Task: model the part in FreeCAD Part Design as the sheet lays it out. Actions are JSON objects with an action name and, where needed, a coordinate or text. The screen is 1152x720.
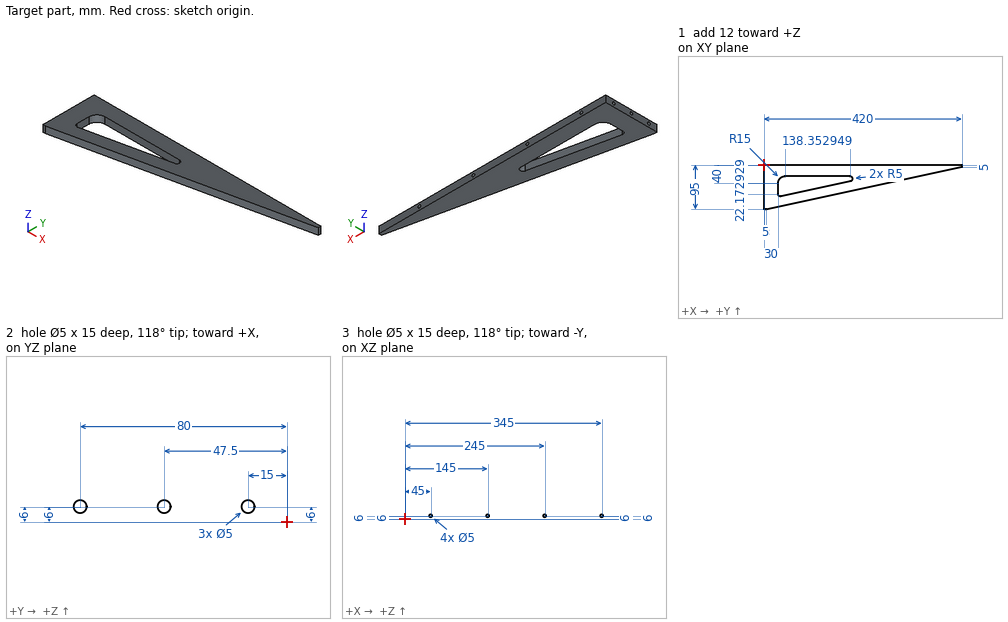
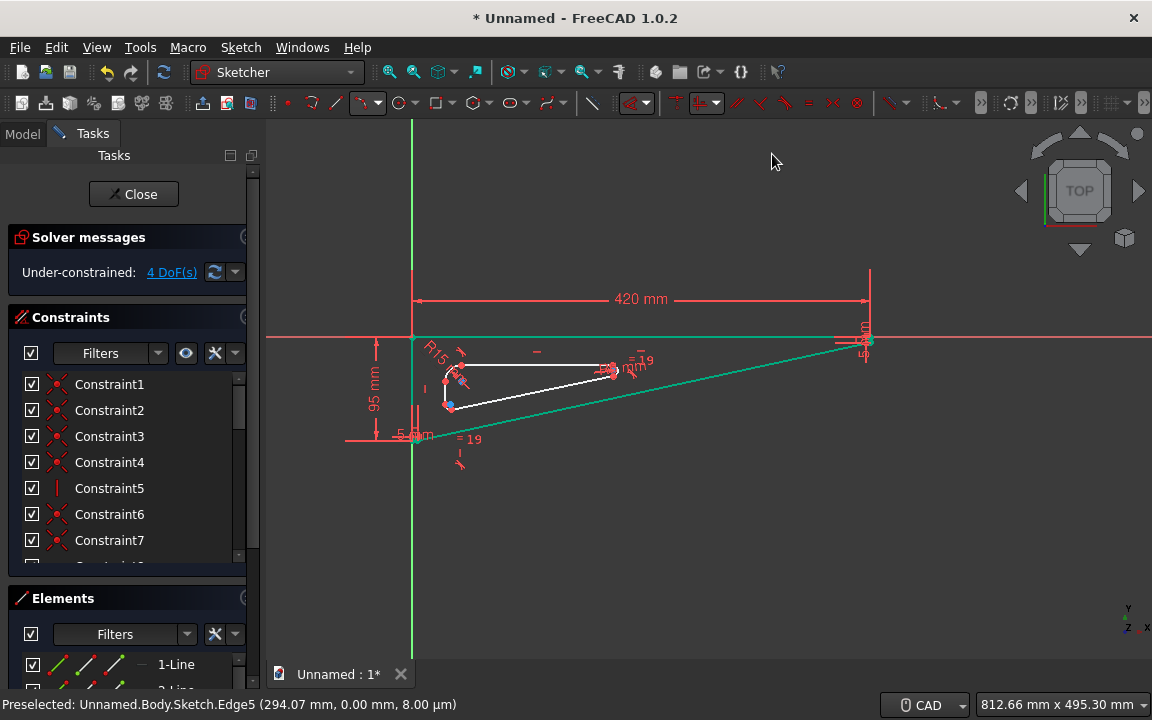
{"action": "scroll", "coordinate": [445, 405], "scroll_direction": "up", "scroll_amount": 5}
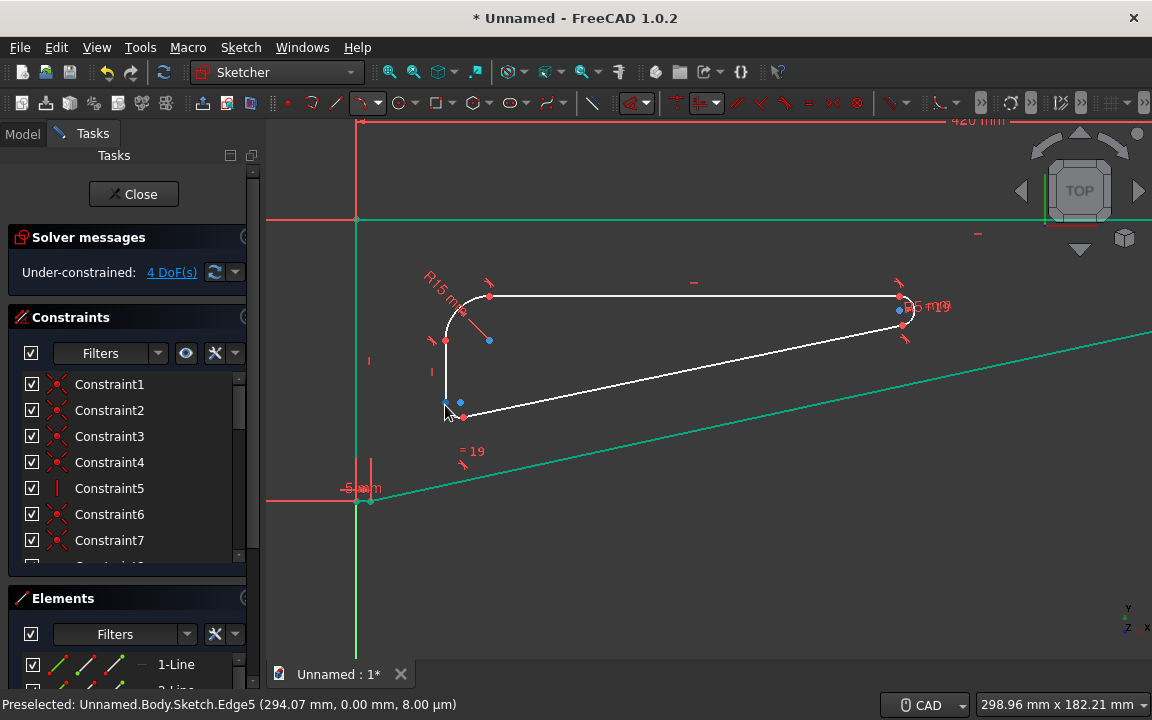
{"action": "left_click", "coordinate": [446, 403]}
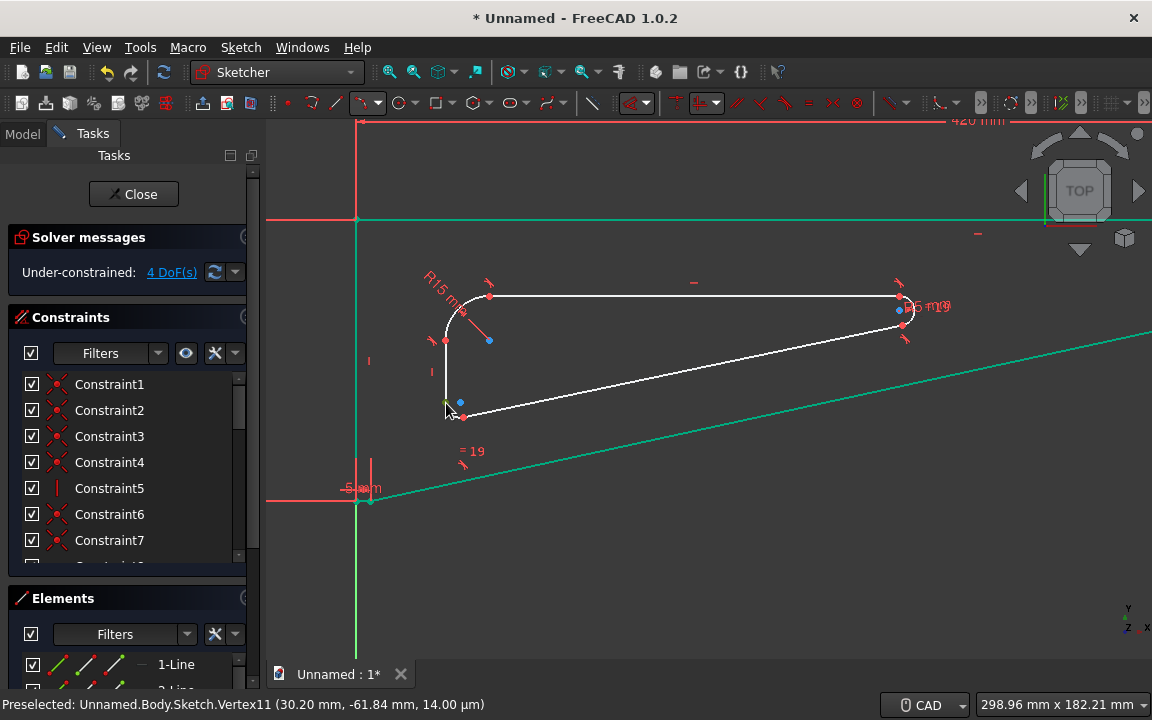
{"action": "left_click", "coordinate": [648, 104]}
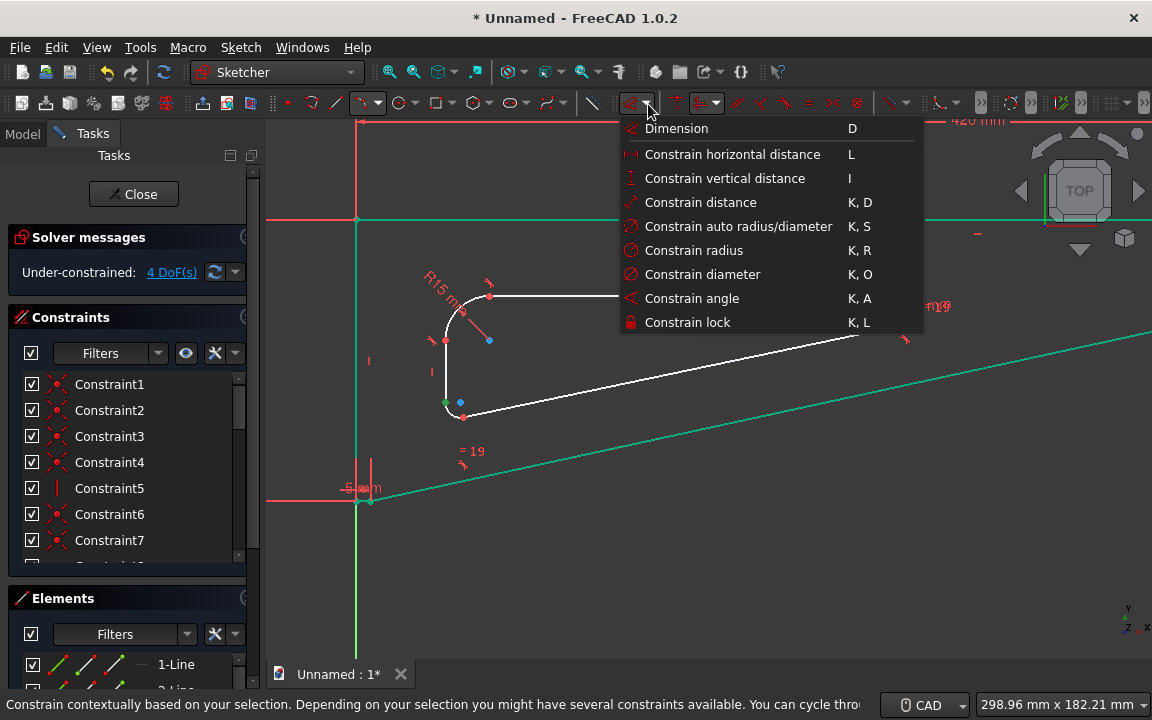
{"action": "left_click", "coordinate": [772, 154]}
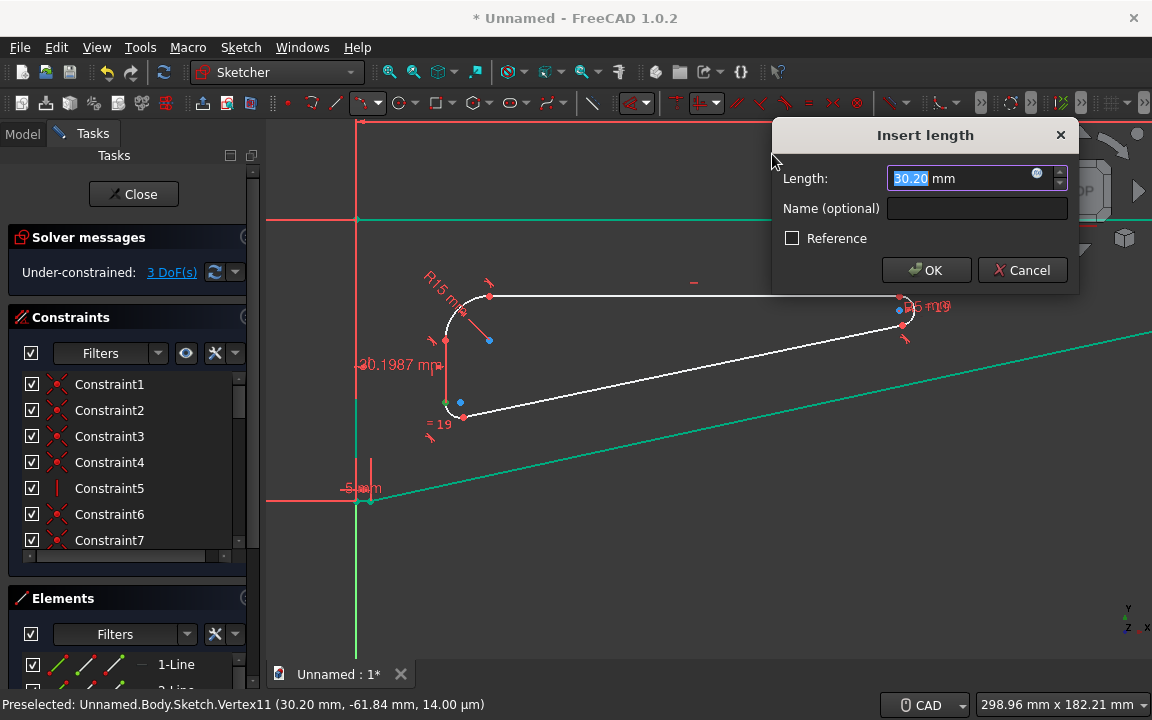
{"action": "type", "text": "30"}
{"action": "key", "text": "Return"}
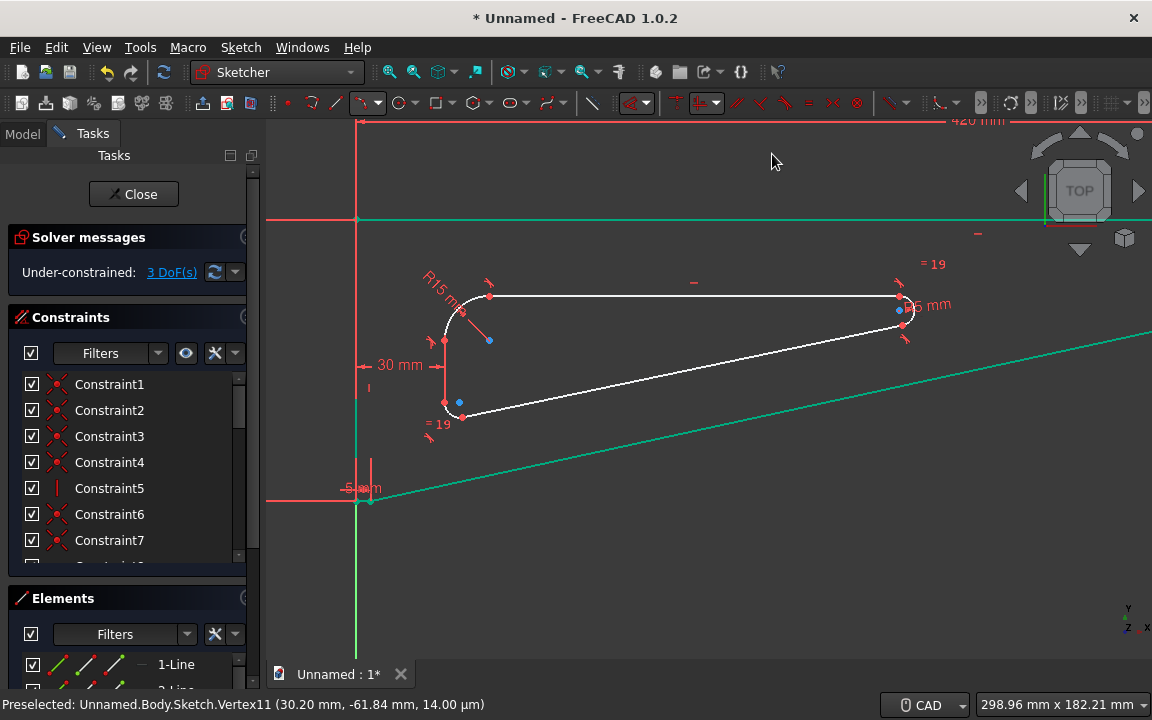
{"action": "left_click", "coordinate": [445, 340]}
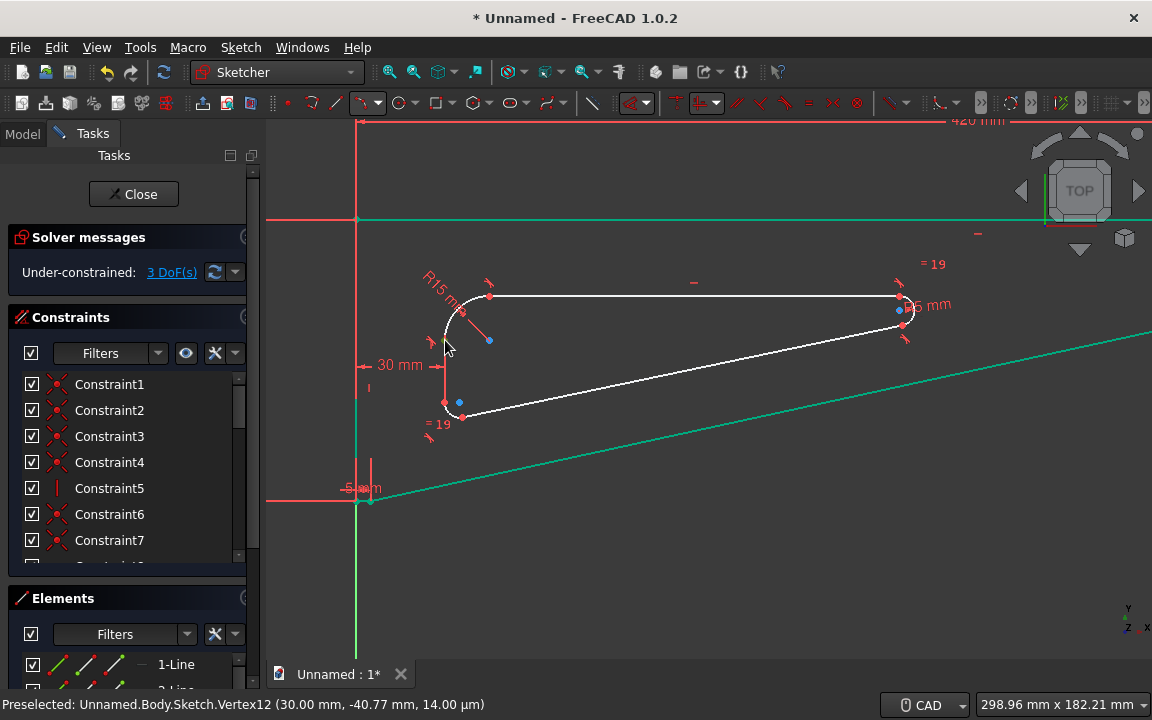
{"action": "key", "text": "i"}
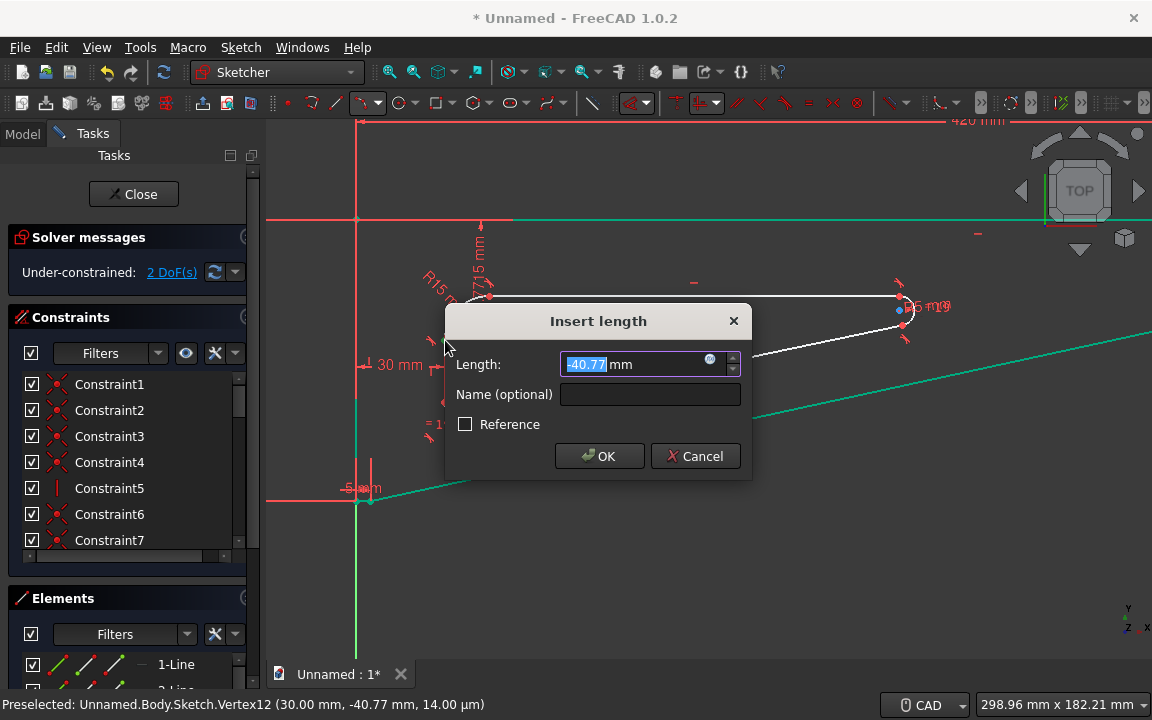
{"action": "type", "text": "-40"}
{"action": "key", "text": "Return"}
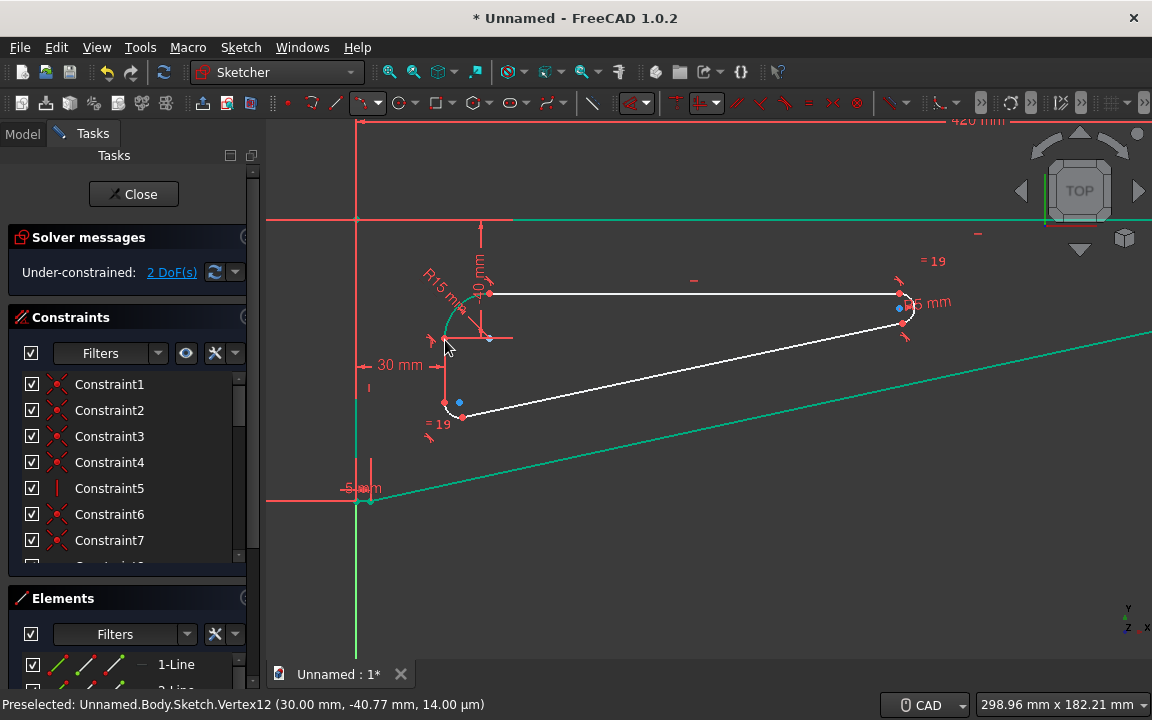
{"action": "left_click", "coordinate": [445, 383]}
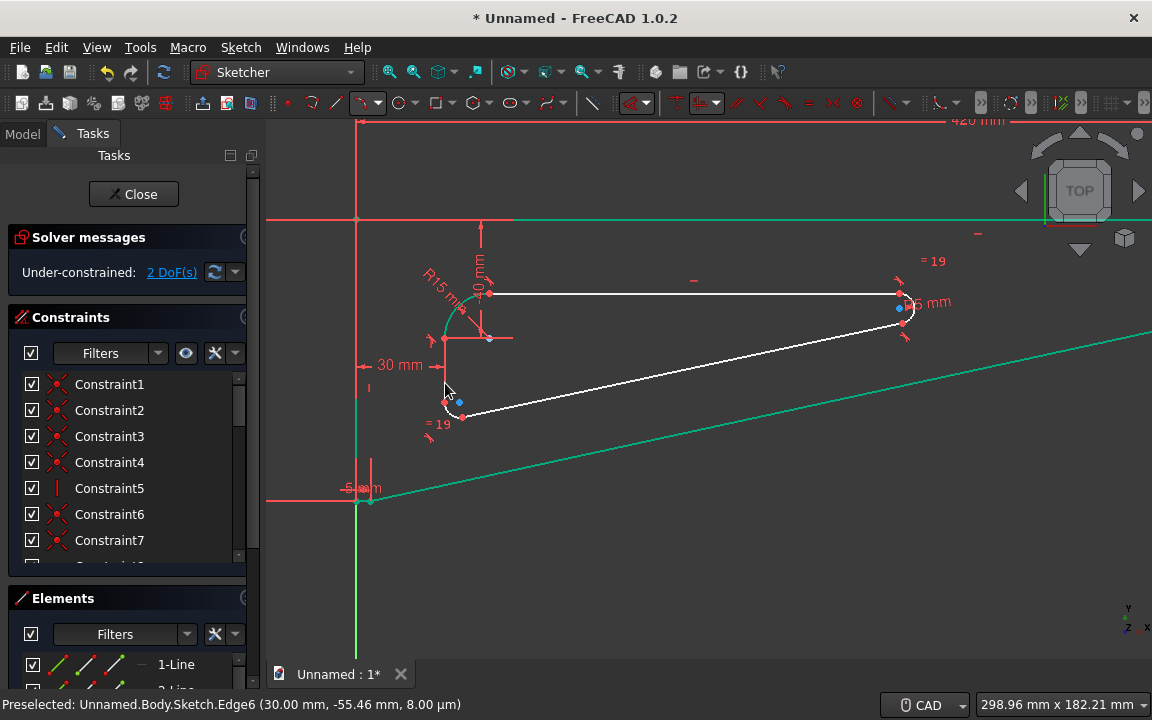
{"action": "left_click", "coordinate": [648, 104]}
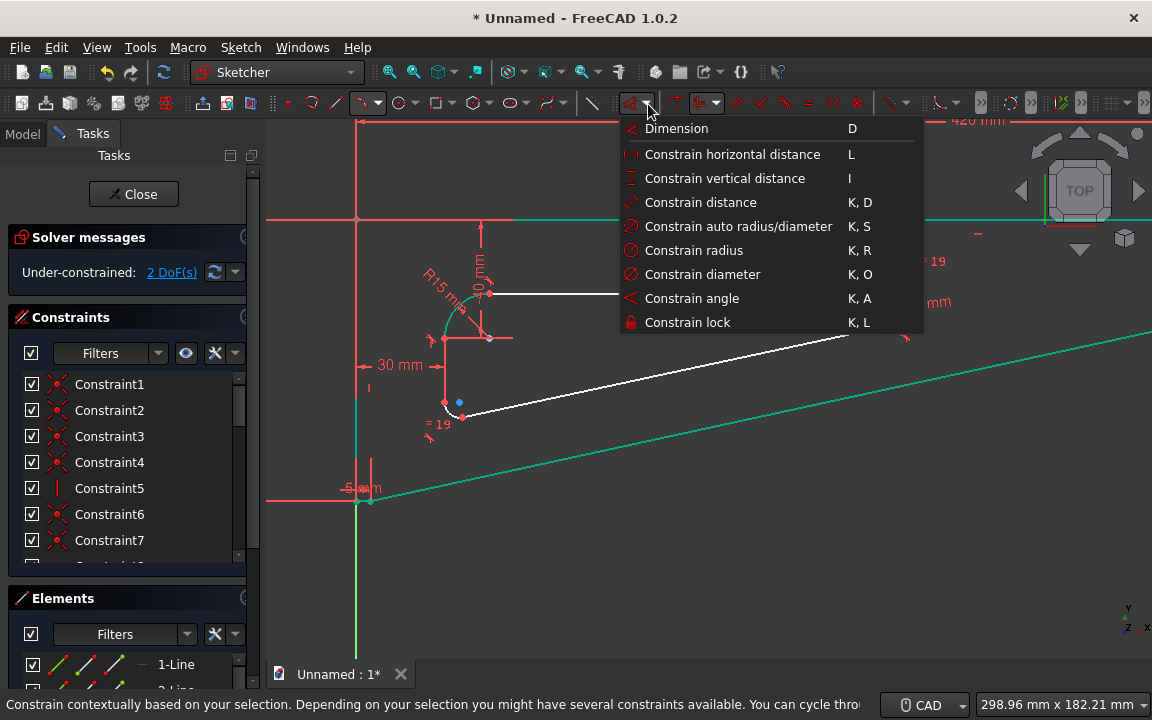
{"action": "left_click", "coordinate": [772, 178]}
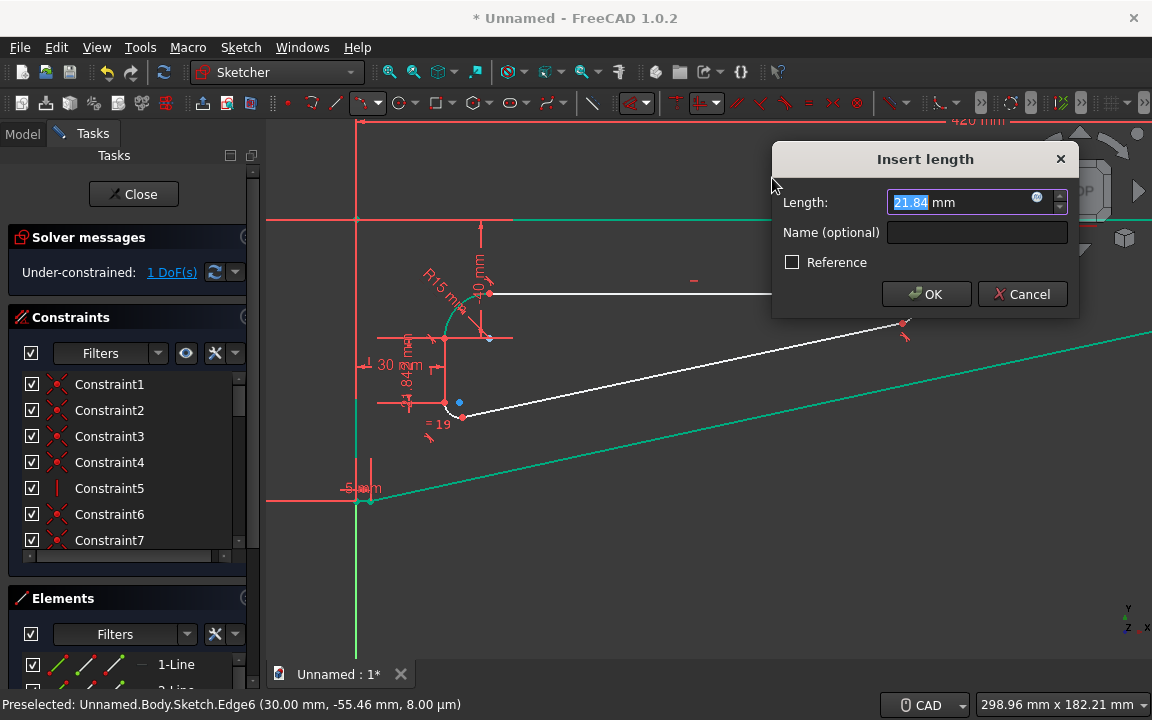
{"action": "type", "text": "22.172929"}
{"action": "key", "text": "Return"}